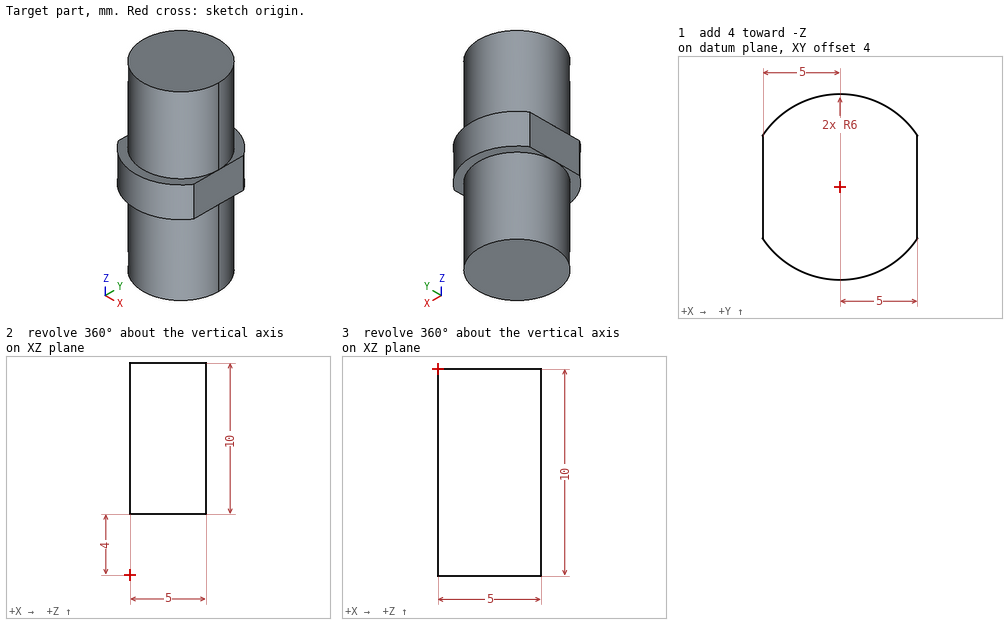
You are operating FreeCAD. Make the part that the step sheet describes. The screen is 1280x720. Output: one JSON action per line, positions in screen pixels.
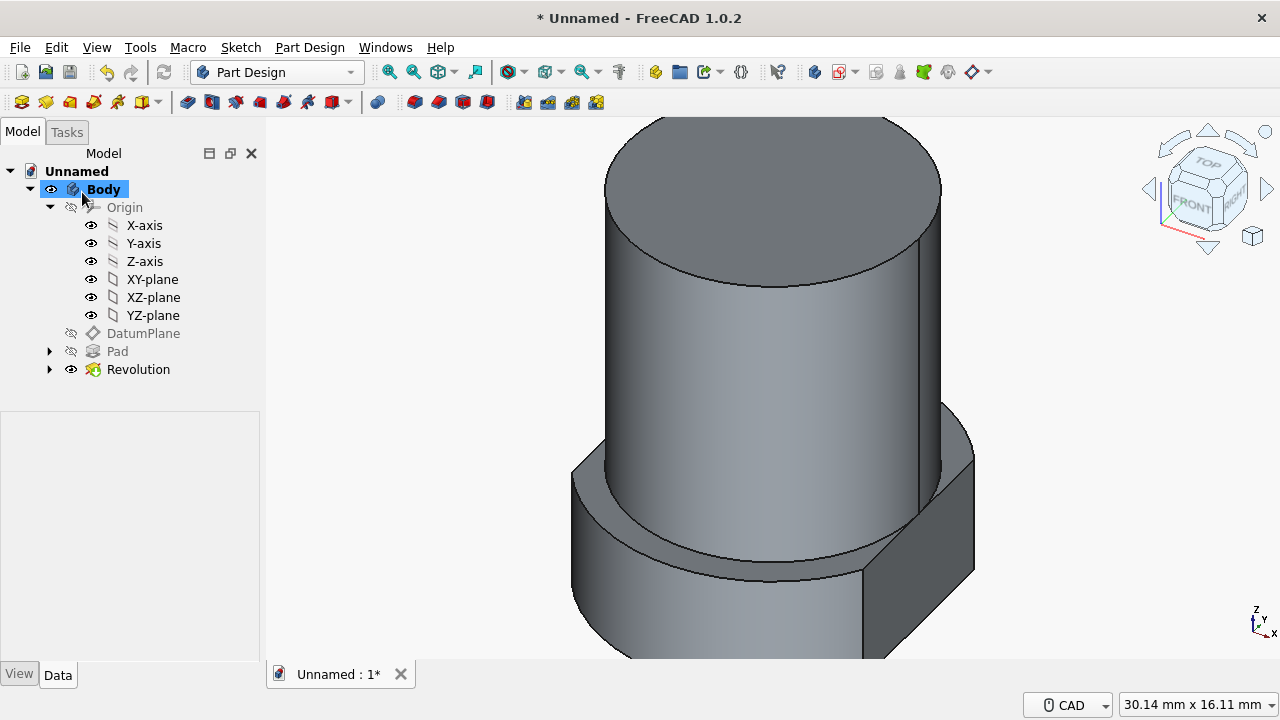
{"action": "left_click", "coordinate": [390, 72]}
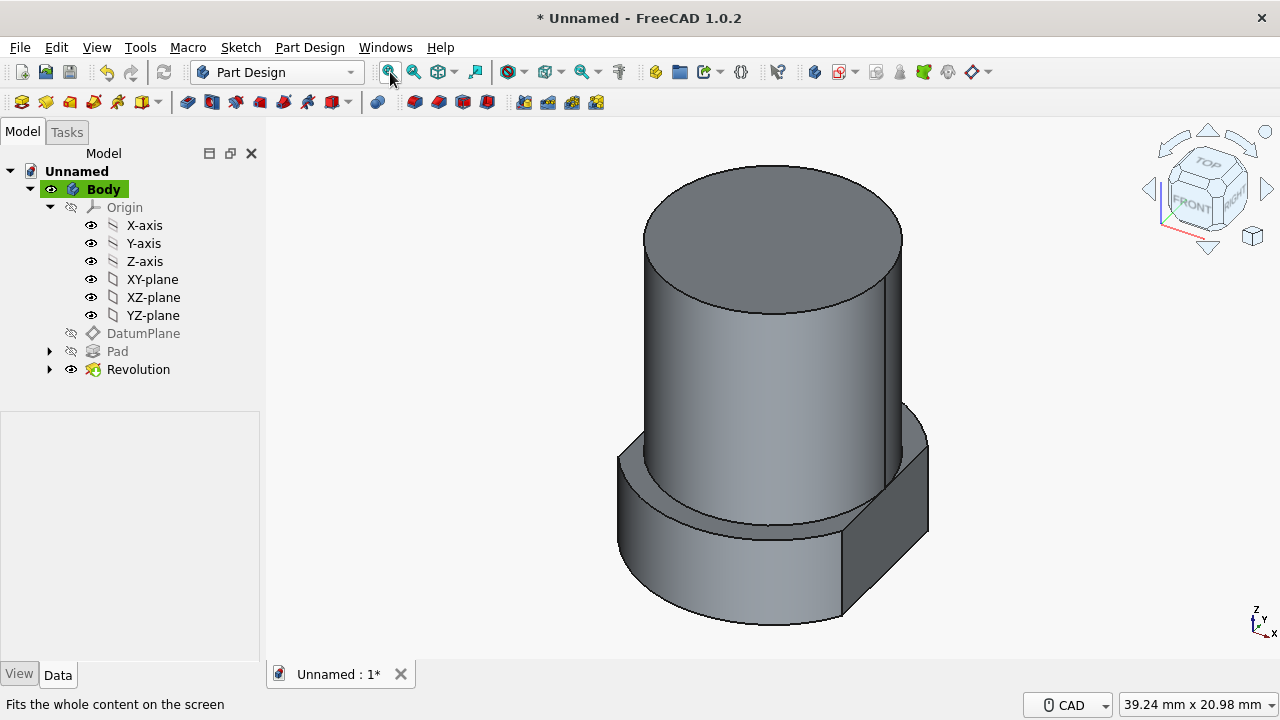
{"action": "left_click", "coordinate": [840, 72]}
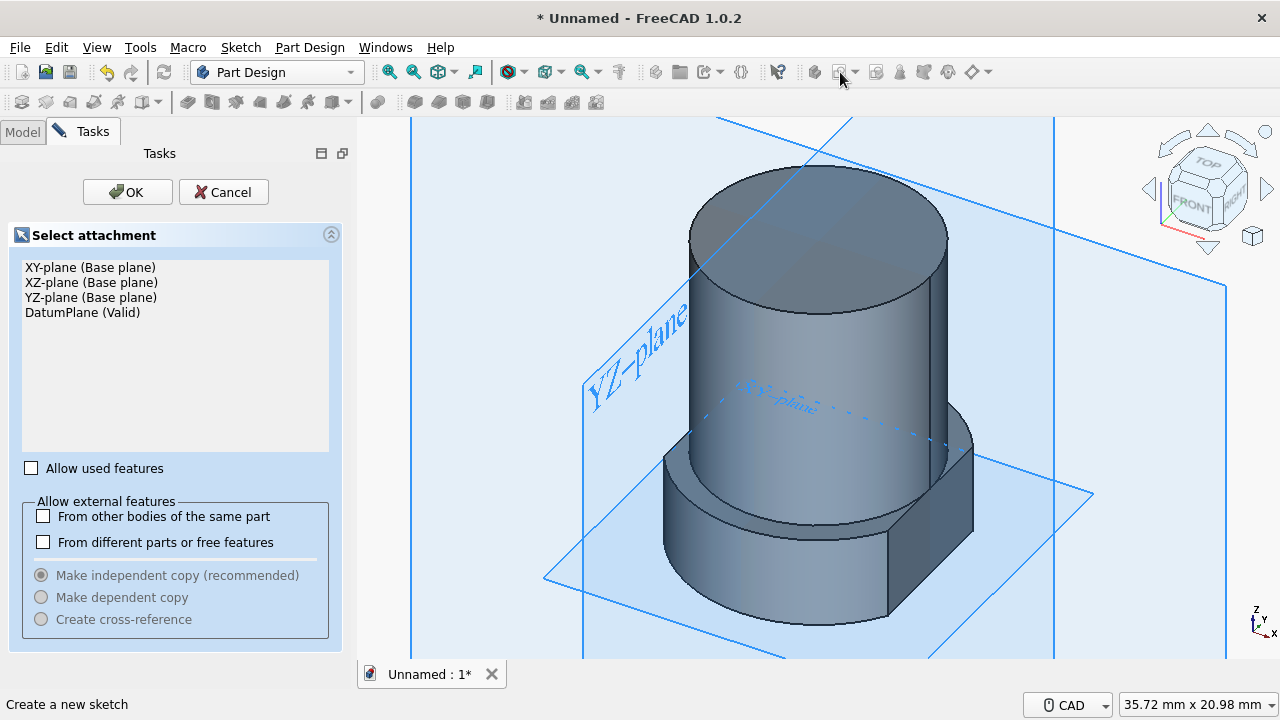
{"action": "left_click", "coordinate": [82, 282]}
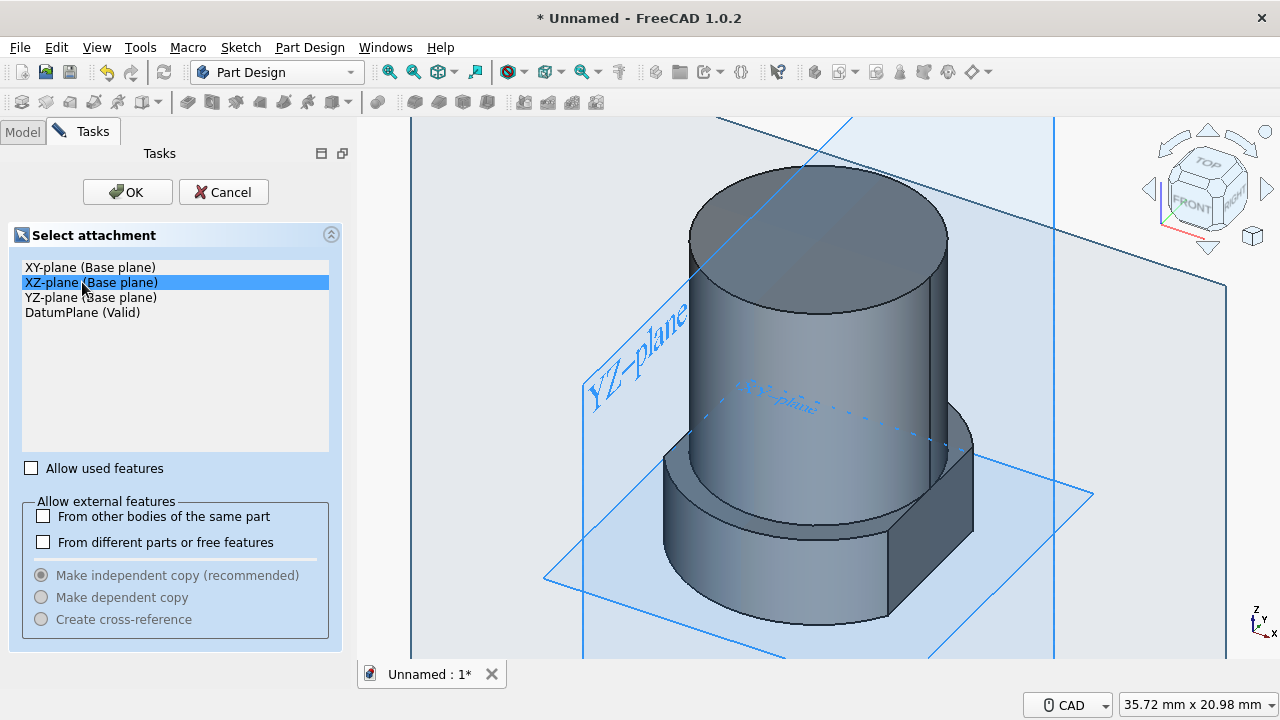
{"action": "left_click", "coordinate": [128, 192]}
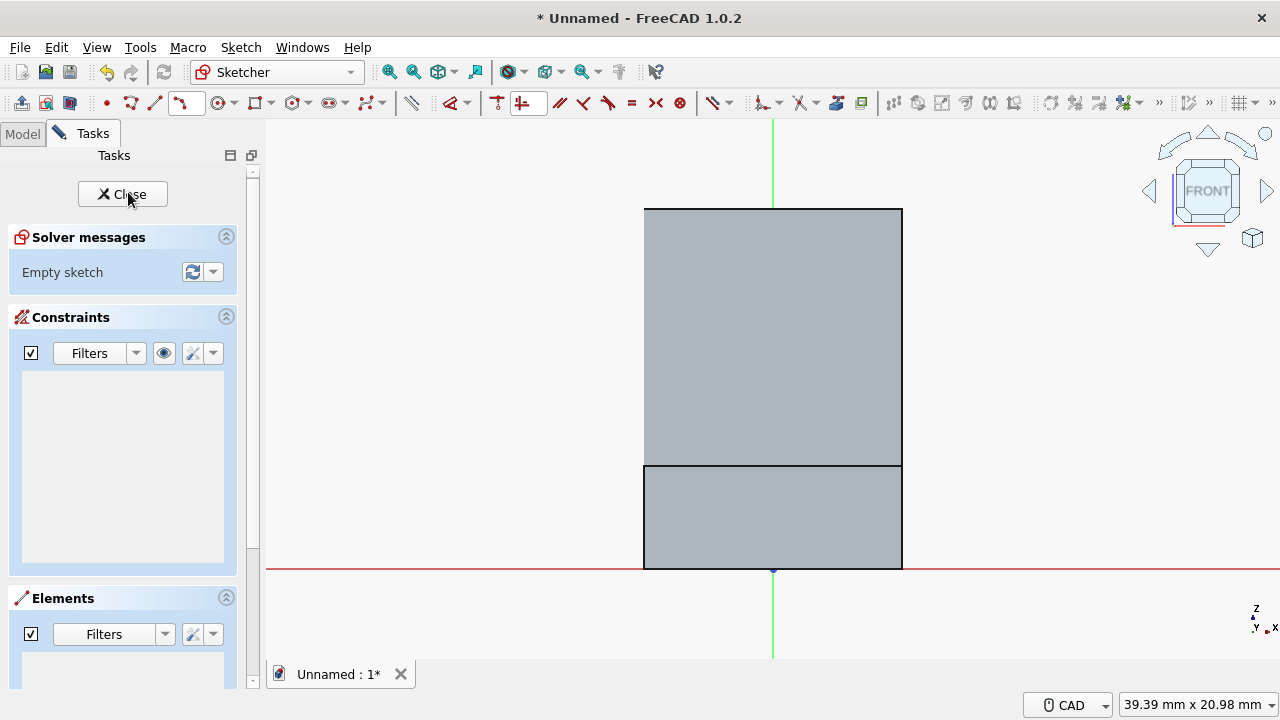
{"action": "left_click", "coordinate": [70, 104]}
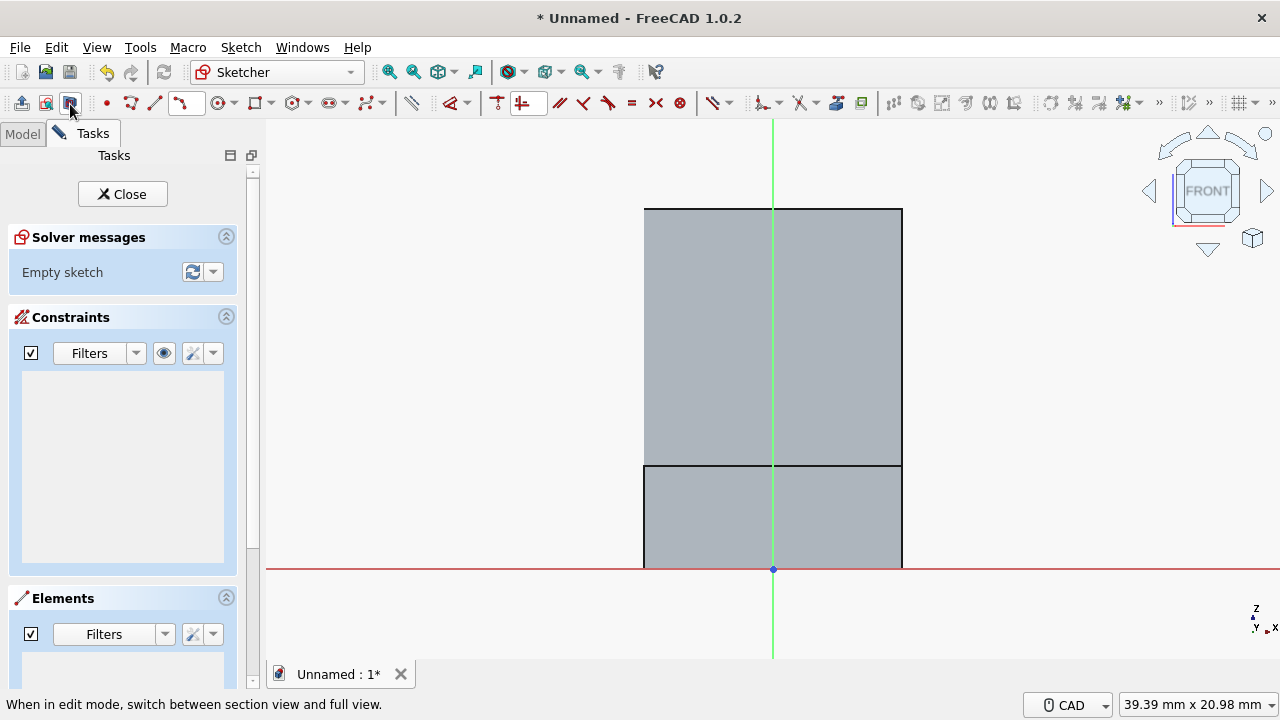
{"action": "scroll", "coordinate": [434, 147], "scroll_direction": "down", "scroll_amount": 2}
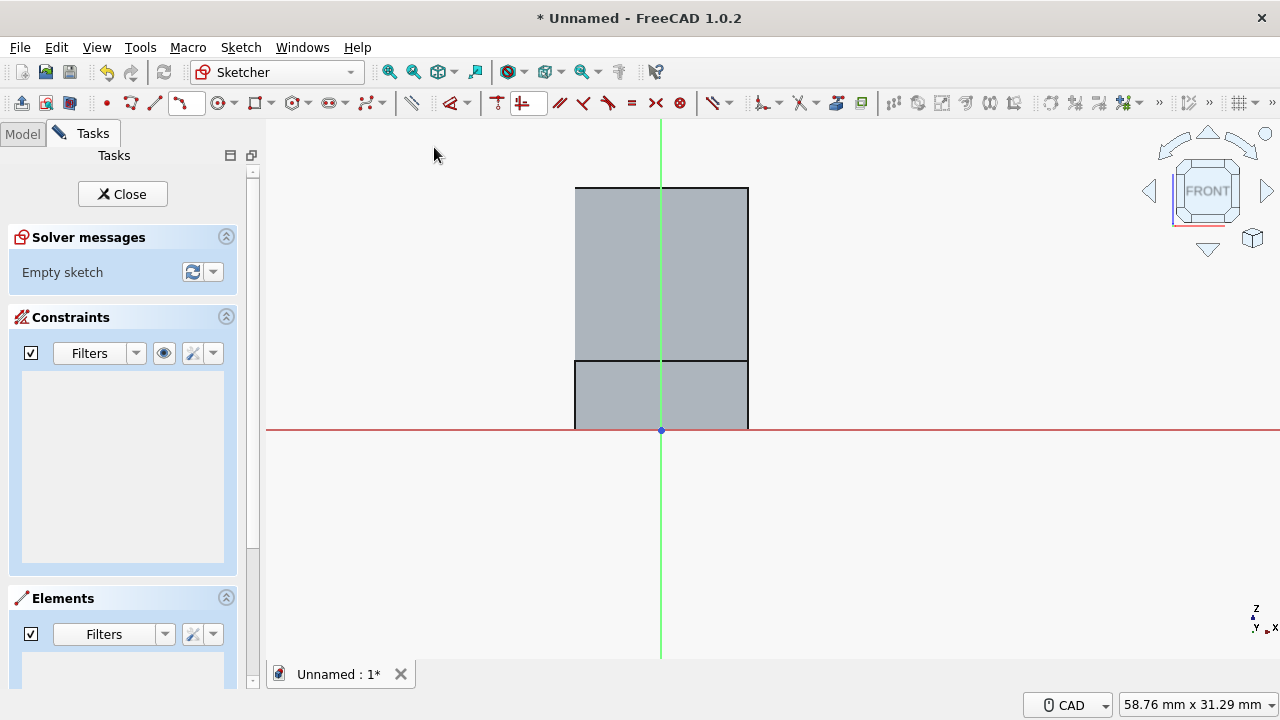
{"action": "scroll", "coordinate": [704, 631], "scroll_direction": "up", "scroll_amount": 3}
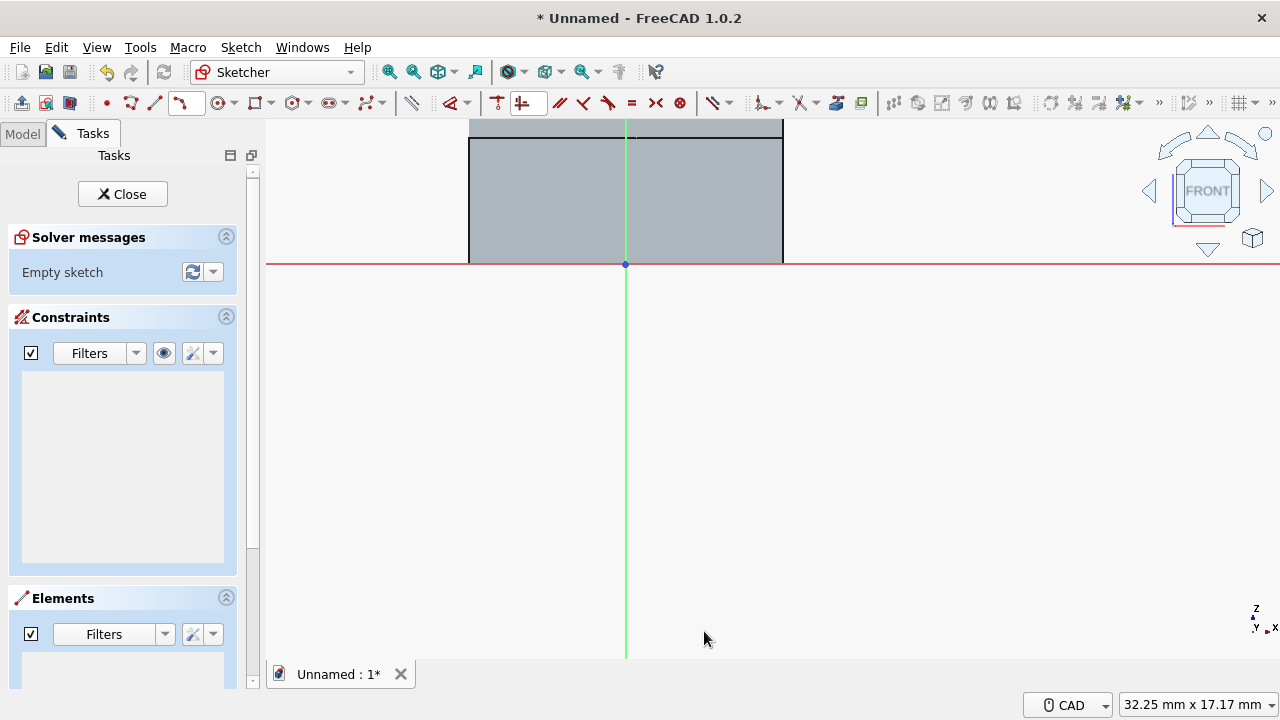
{"action": "left_click", "coordinate": [256, 104]}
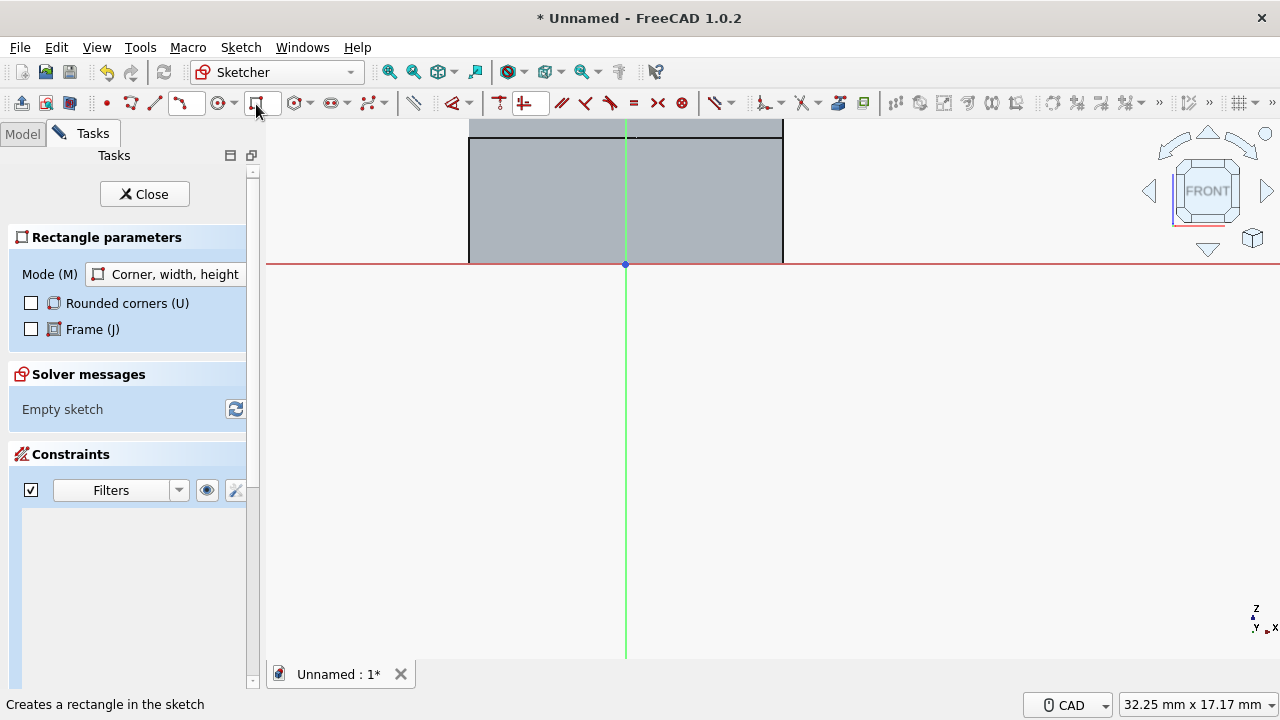
{"action": "left_click", "coordinate": [626, 264]}
{"action": "mouse_move", "coordinate": [783, 578]}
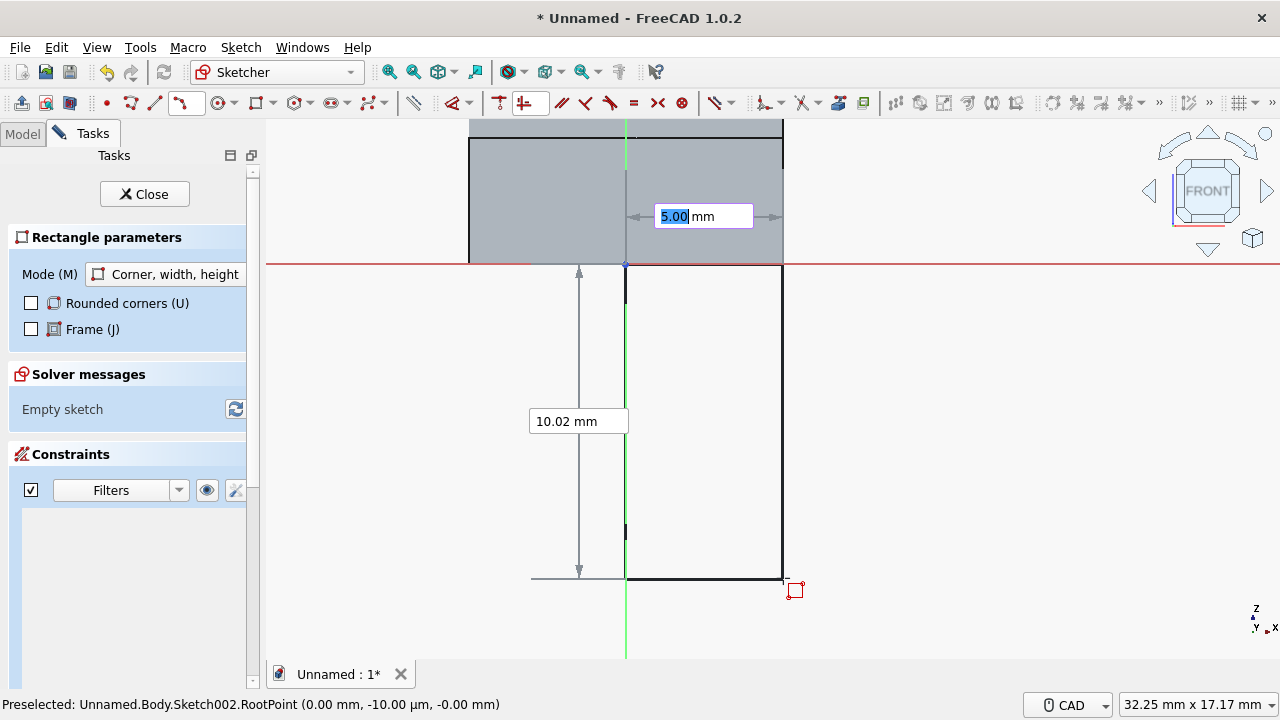
{"action": "type", "text": "5"}
{"action": "key", "text": "Tab"}
{"action": "type", "text": "10"}
{"action": "key", "text": "Return"}
{"action": "key", "text": "Escape"}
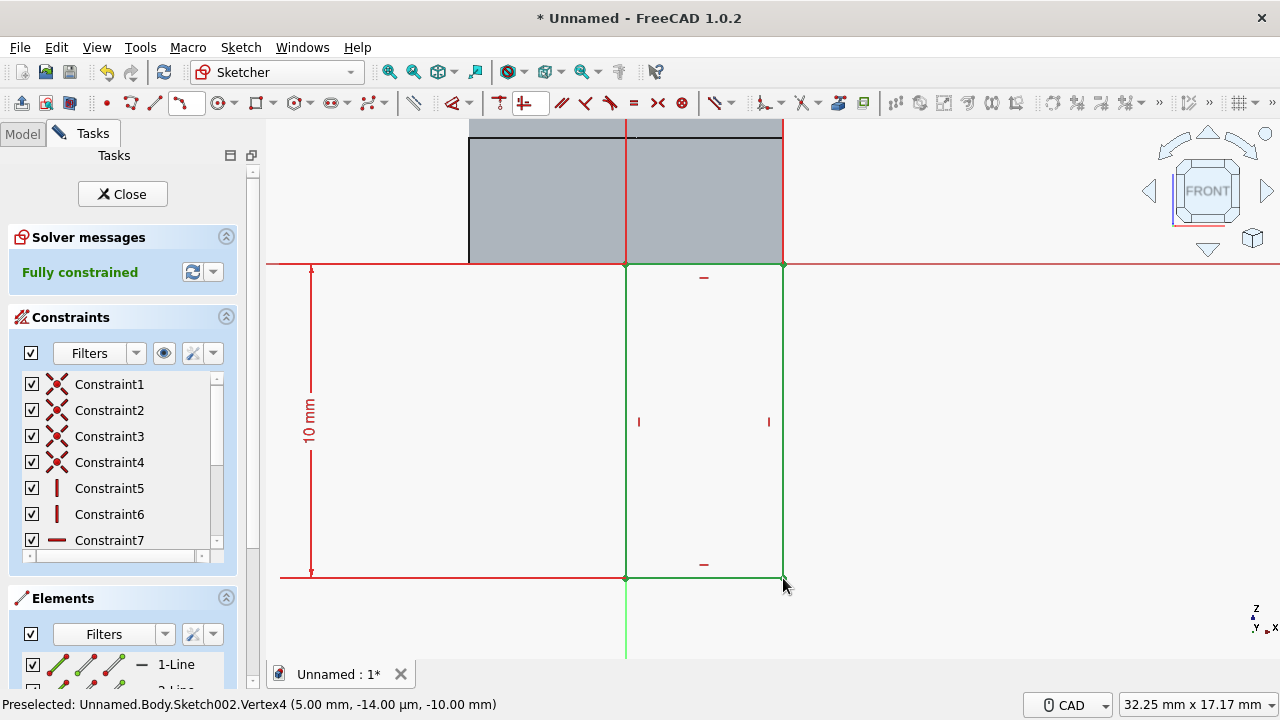
{"action": "left_click", "coordinate": [123, 194]}